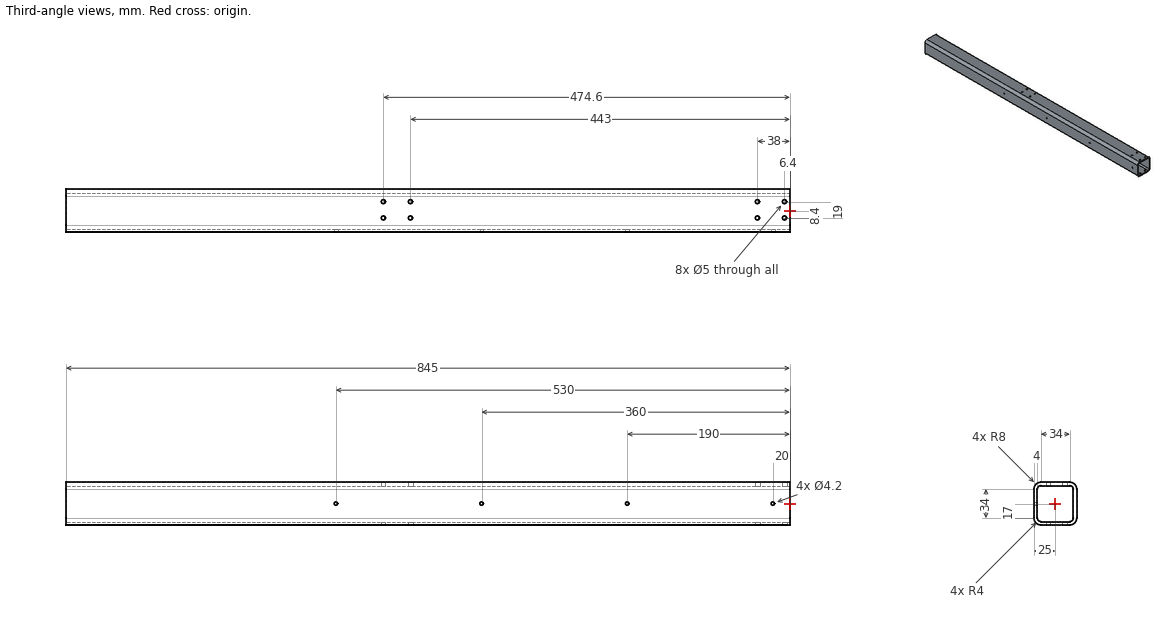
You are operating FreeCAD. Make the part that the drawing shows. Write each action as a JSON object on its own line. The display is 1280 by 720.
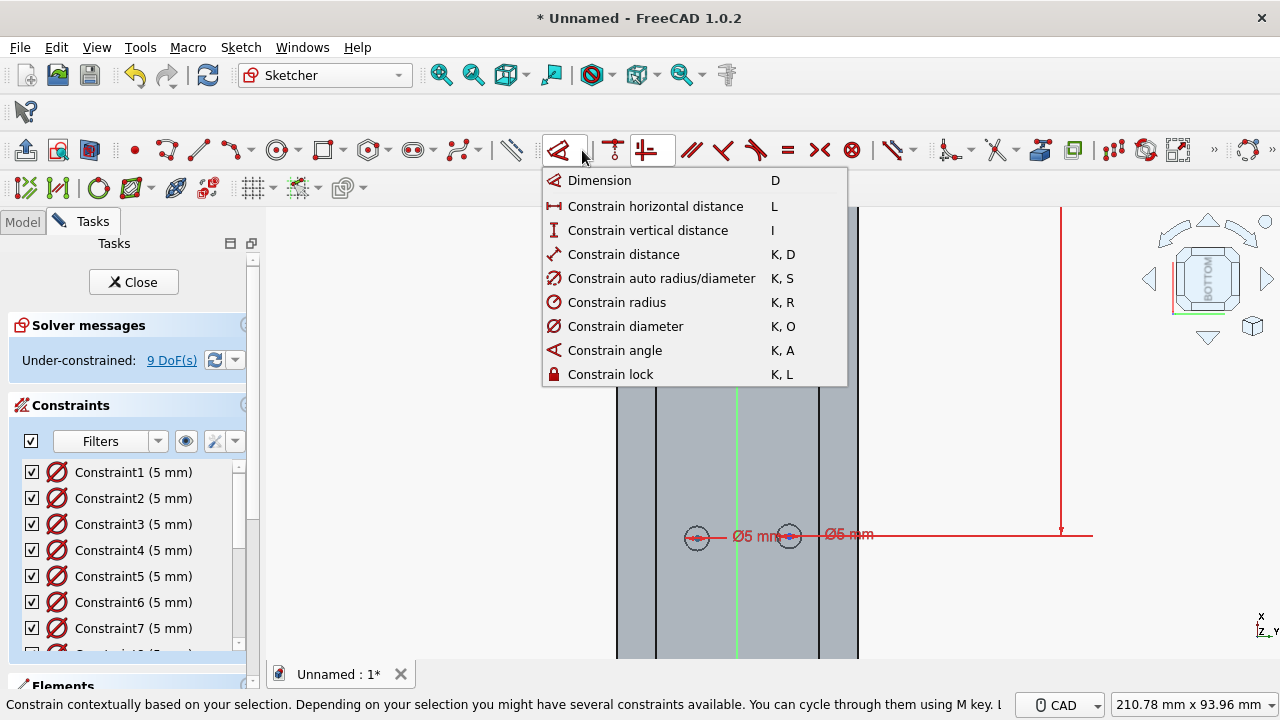
{"action": "left_click", "coordinate": [695, 206]}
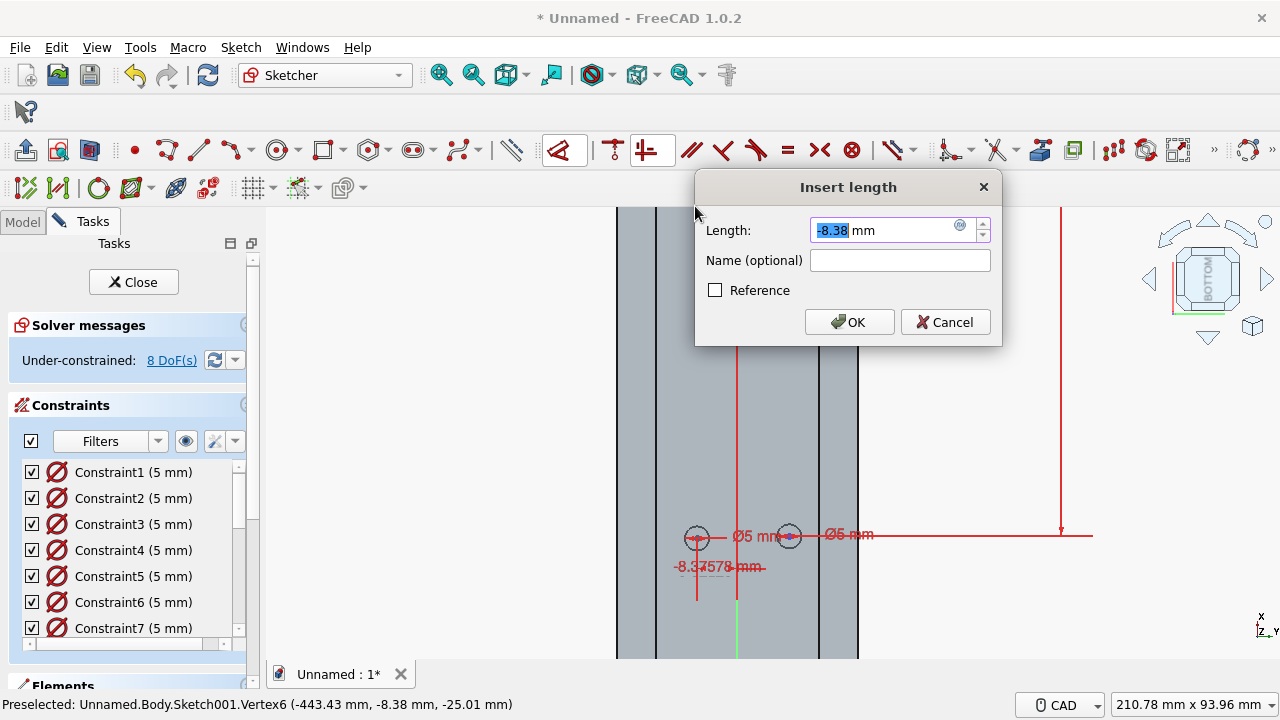
{"action": "type", "text": "-8.4"}
{"action": "key", "text": "Return"}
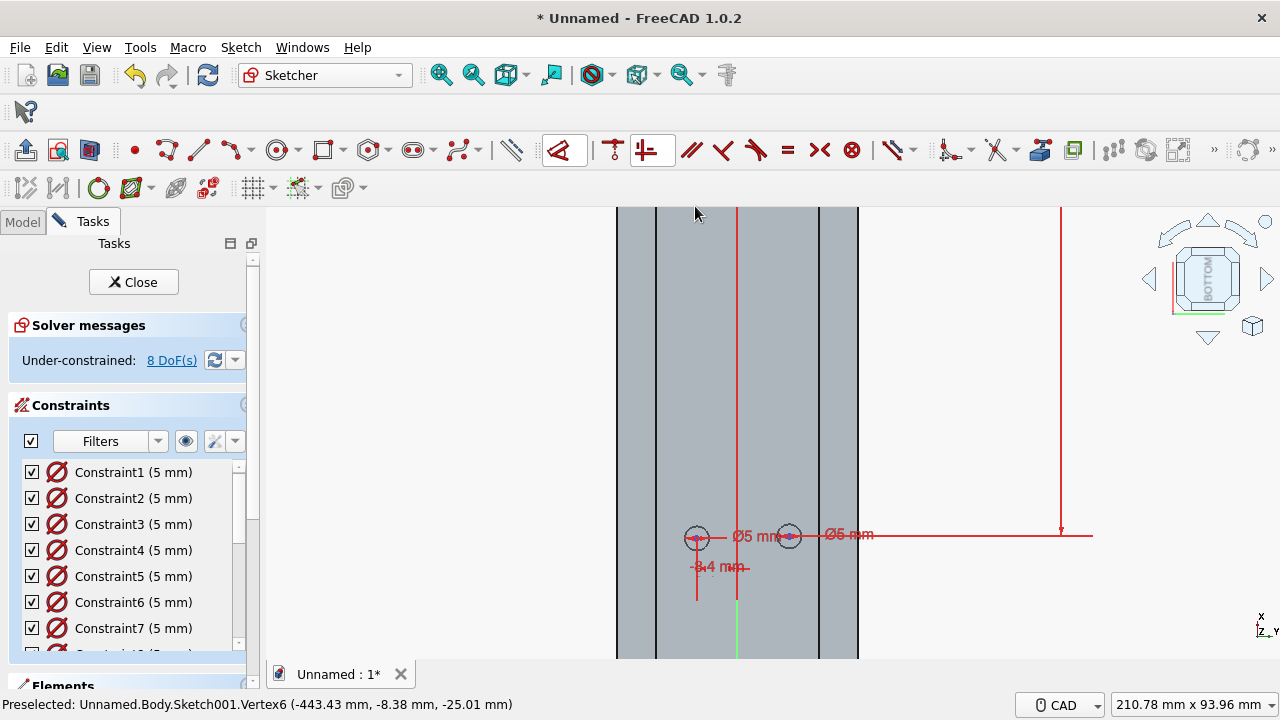
{"action": "scroll", "coordinate": [700, 543], "scroll_direction": "down", "scroll_amount": 11}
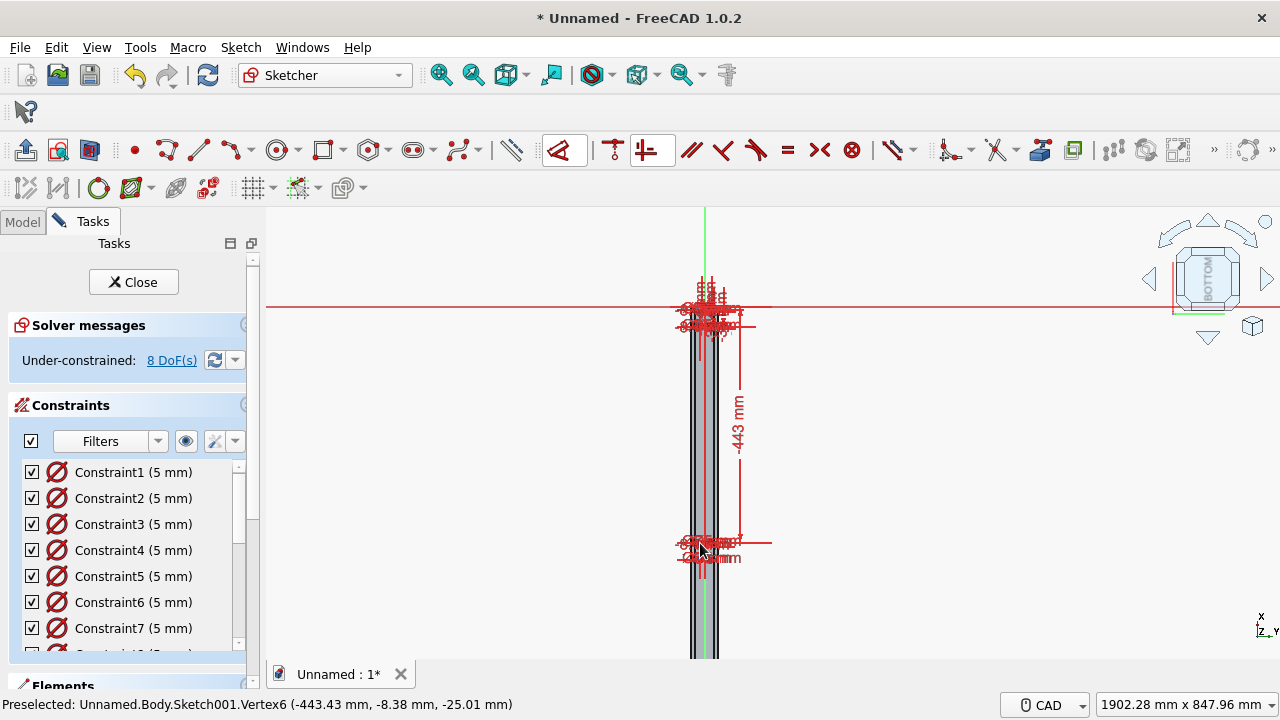
{"action": "left_click", "coordinate": [700, 543]}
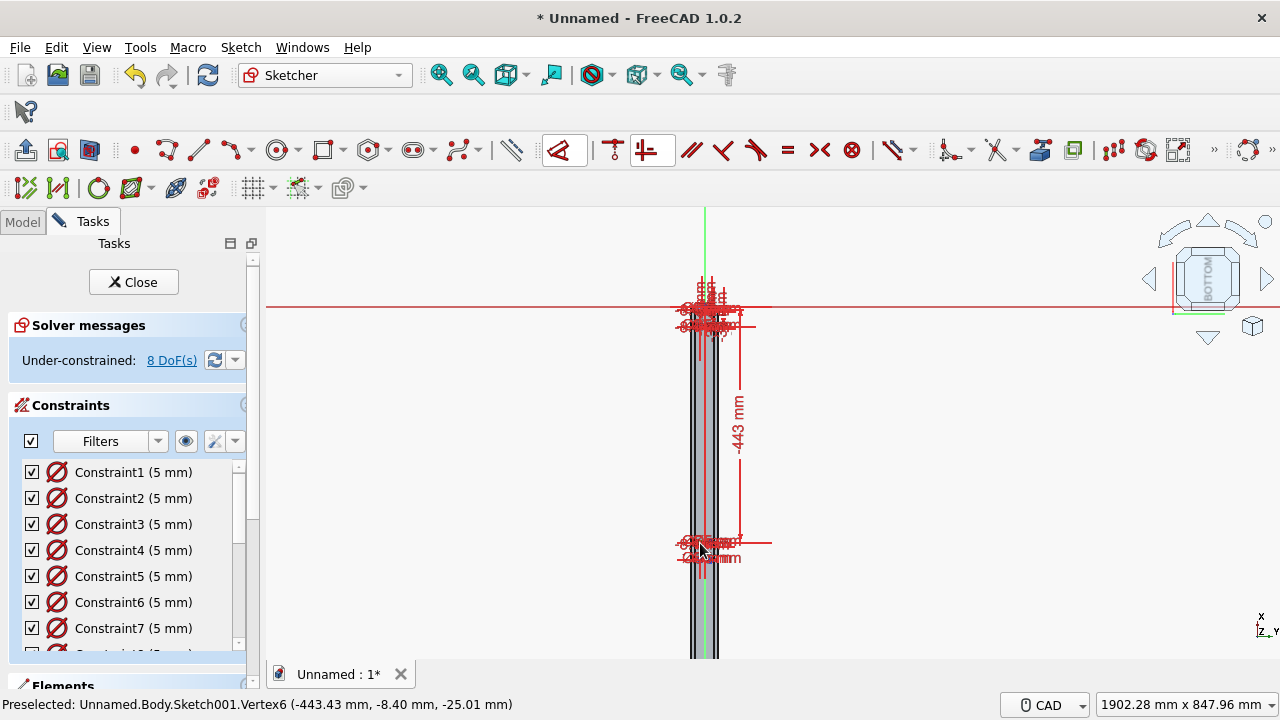
{"action": "key", "text": "i"}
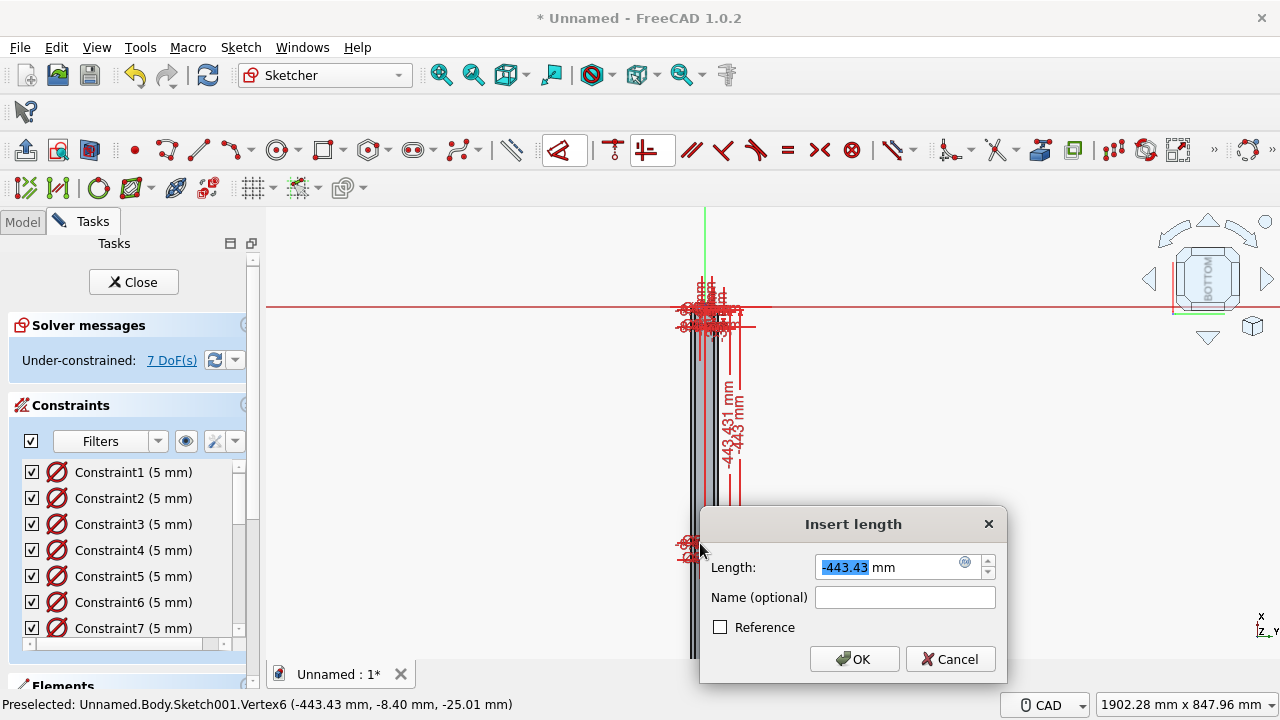
{"action": "type", "text": "-443"}
{"action": "key", "text": "Return"}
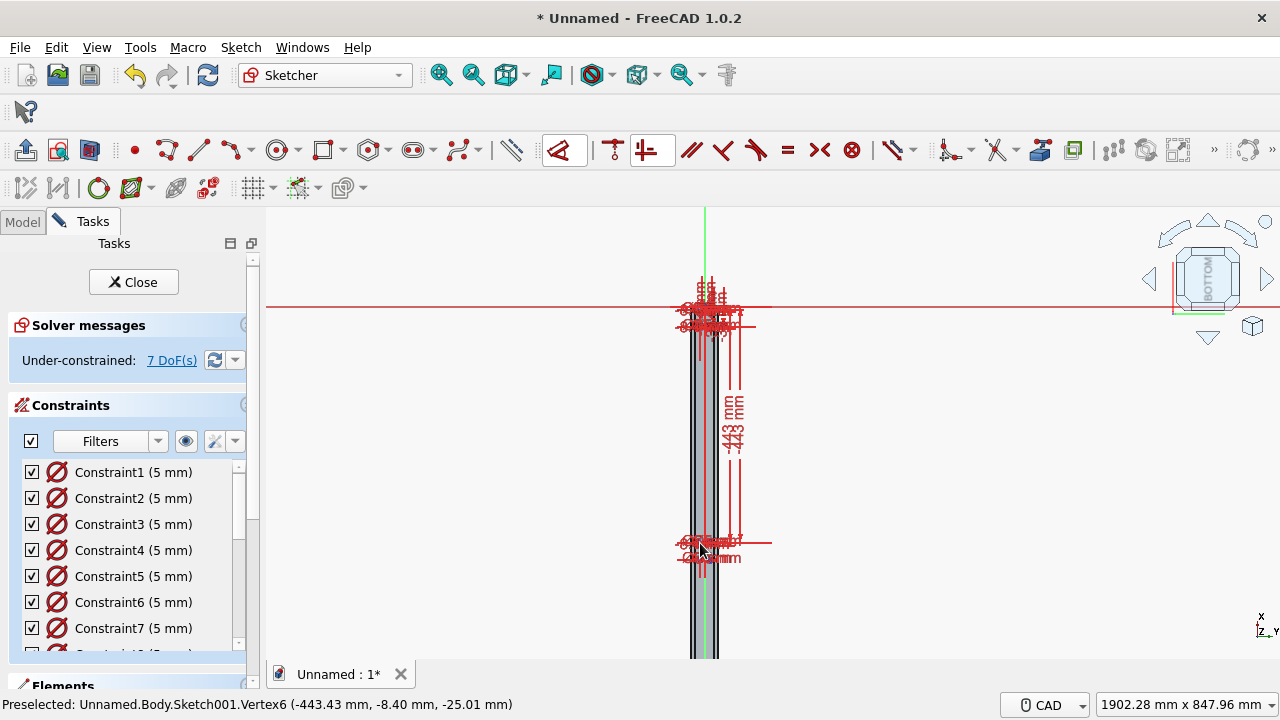
{"action": "scroll", "coordinate": [700, 560], "scroll_direction": "up", "scroll_amount": 11}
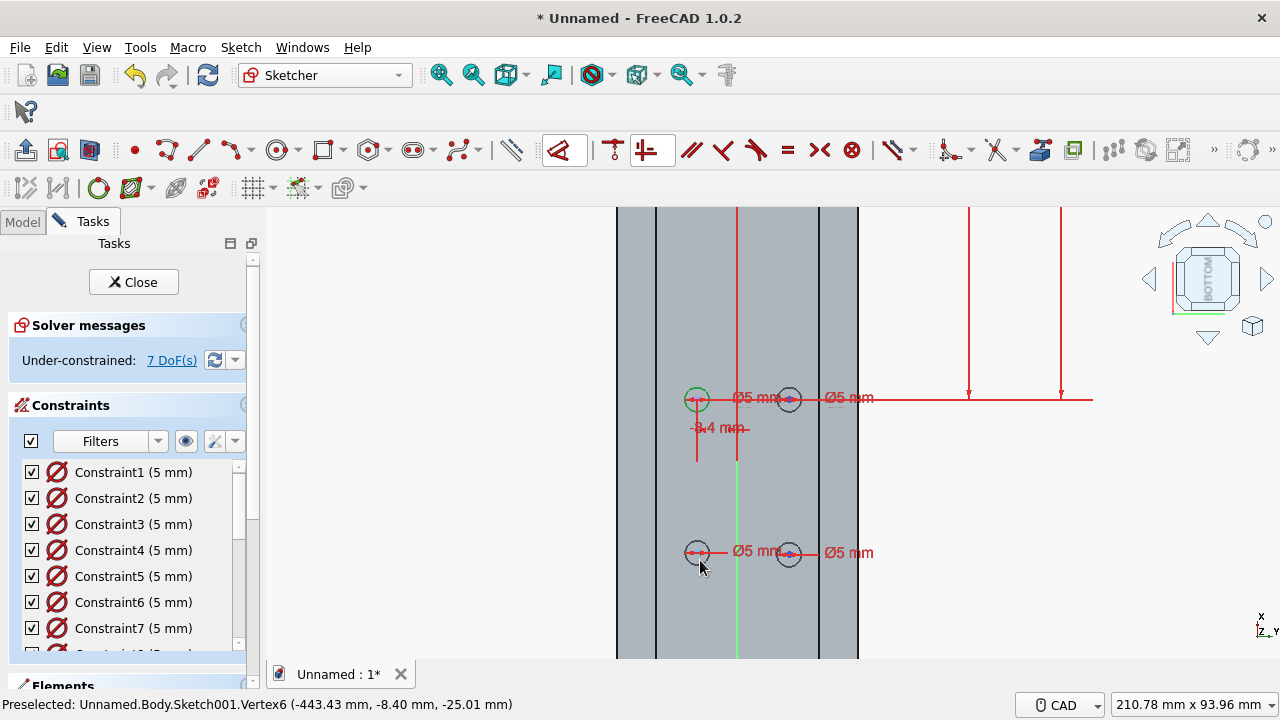
{"action": "left_click", "coordinate": [697, 553]}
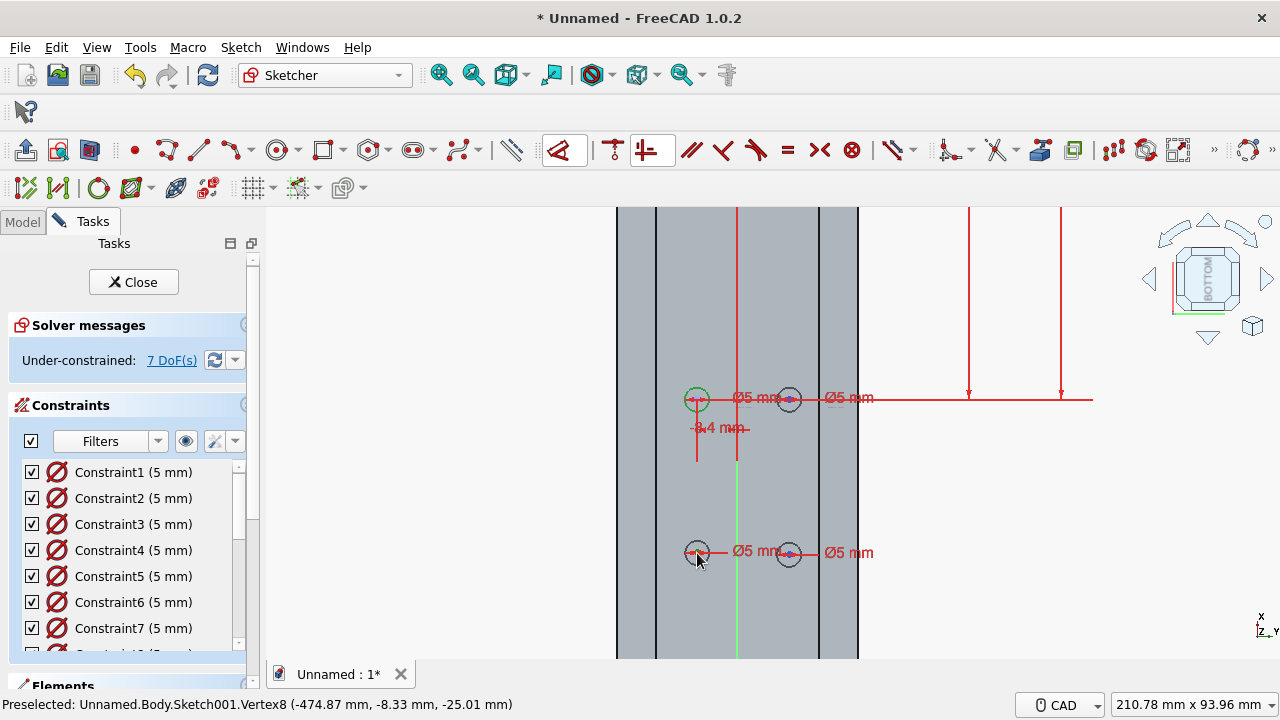
{"action": "key", "text": "l"}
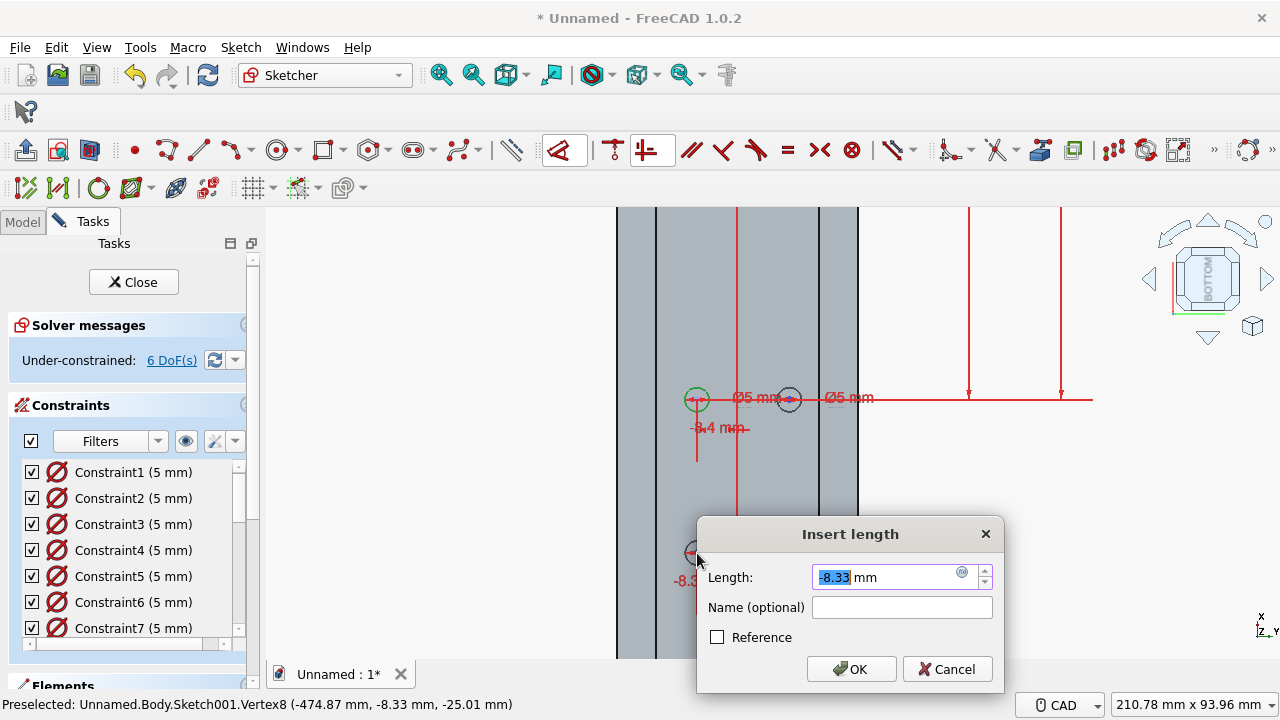
{"action": "type", "text": "-8.4"}
{"action": "key", "text": "Return"}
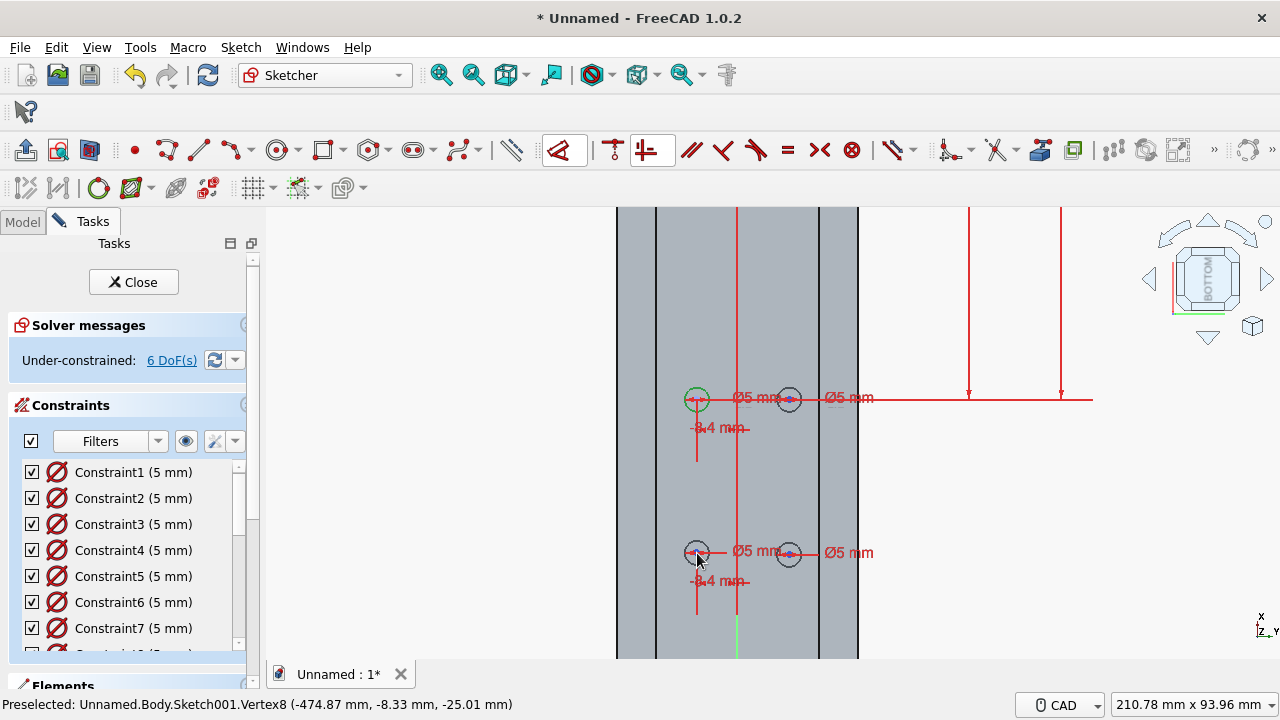
{"action": "scroll", "coordinate": [700, 560], "scroll_direction": "down", "scroll_amount": 11}